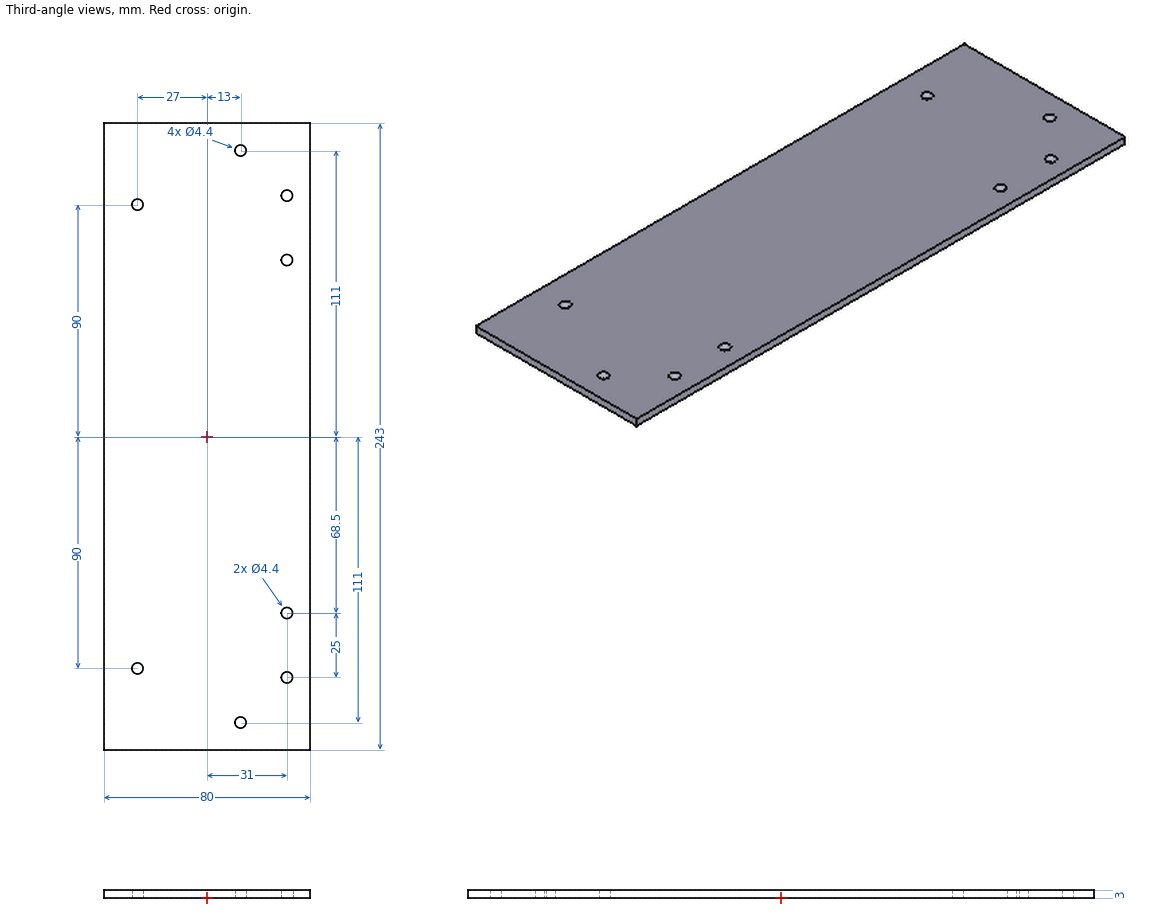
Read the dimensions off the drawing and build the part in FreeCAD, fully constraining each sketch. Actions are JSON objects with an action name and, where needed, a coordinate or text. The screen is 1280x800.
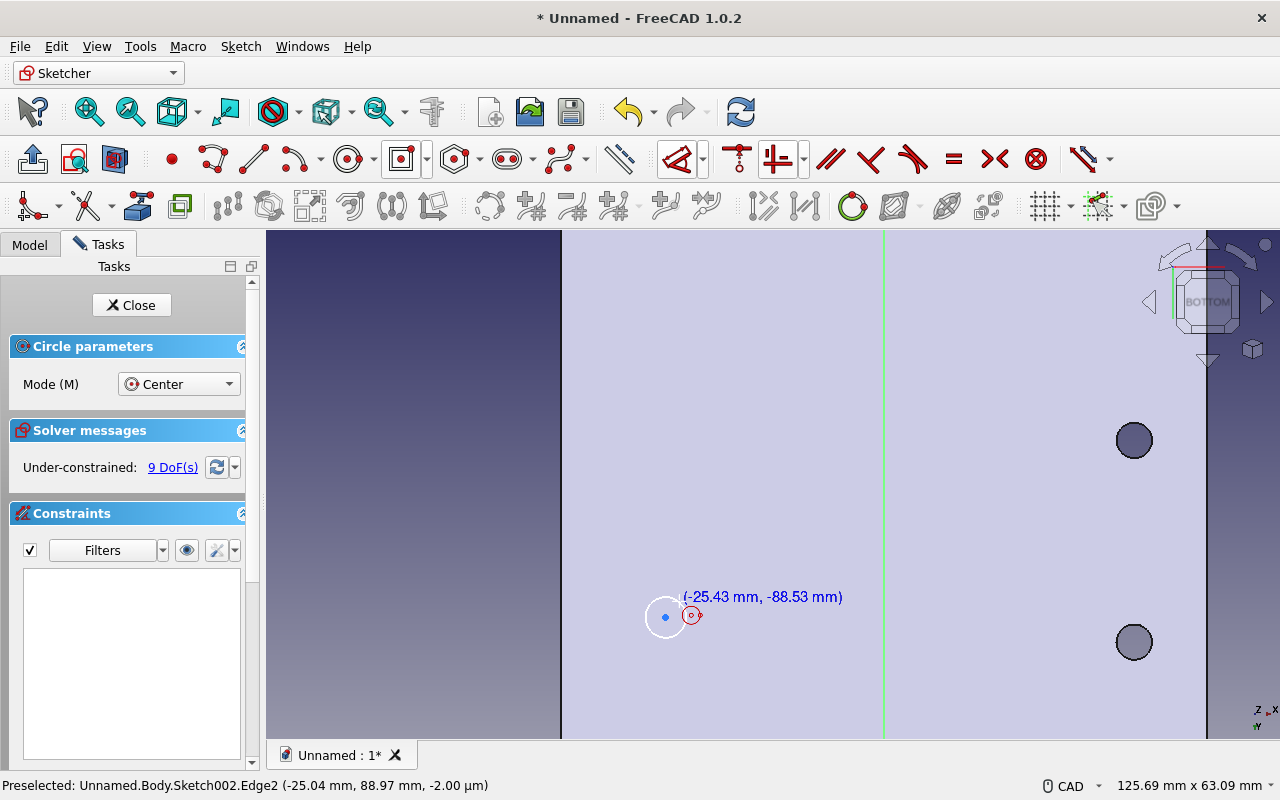
{"action": "scroll", "coordinate": [680, 603], "scroll_direction": "down", "scroll_amount": 9}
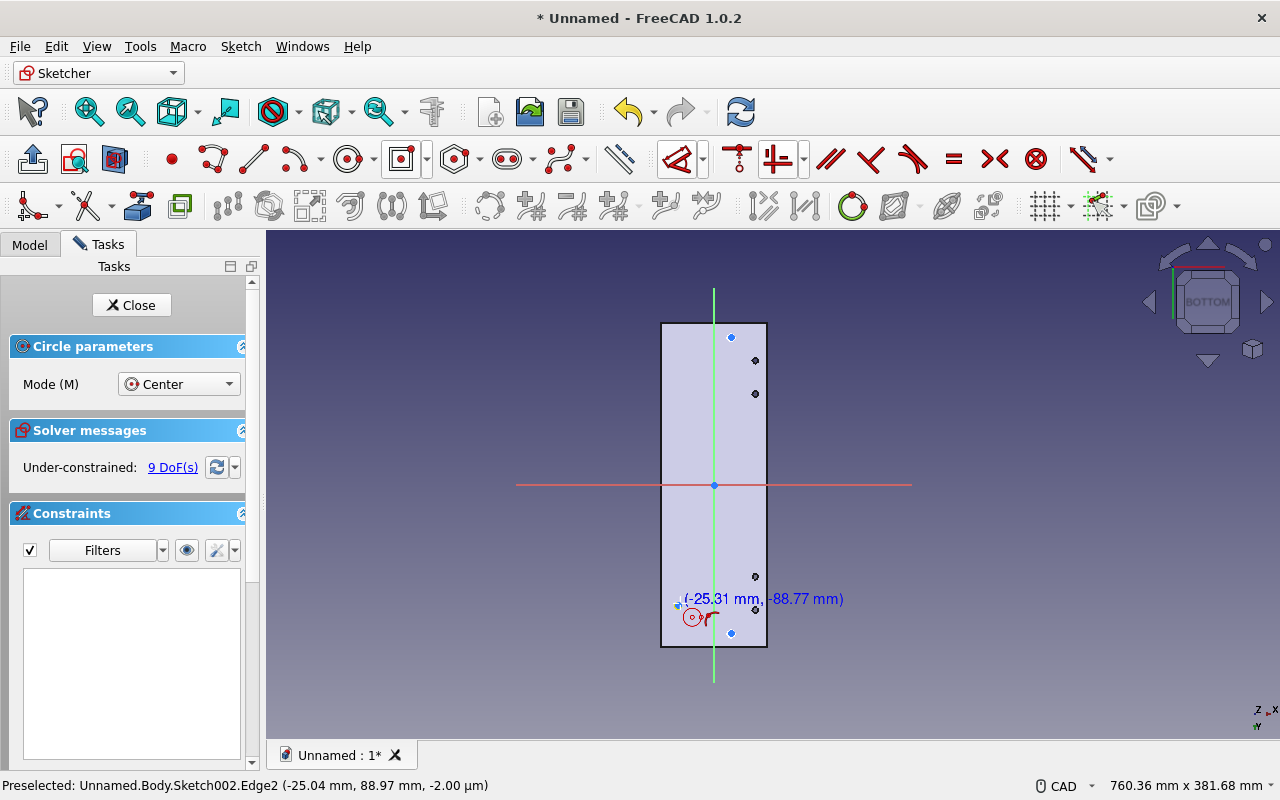
{"action": "scroll", "coordinate": [678, 365], "scroll_direction": "up", "scroll_amount": 11}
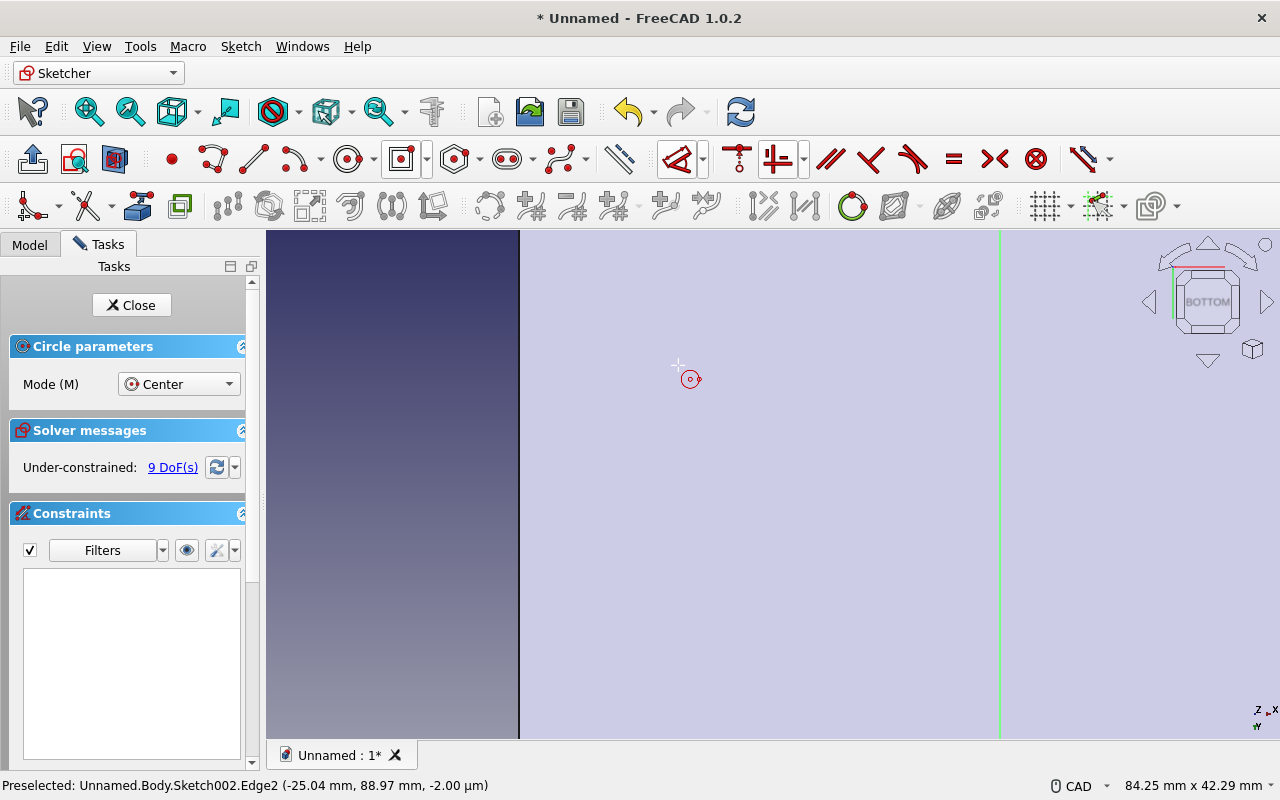
{"action": "scroll", "coordinate": [678, 364], "scroll_direction": "down", "scroll_amount": 11}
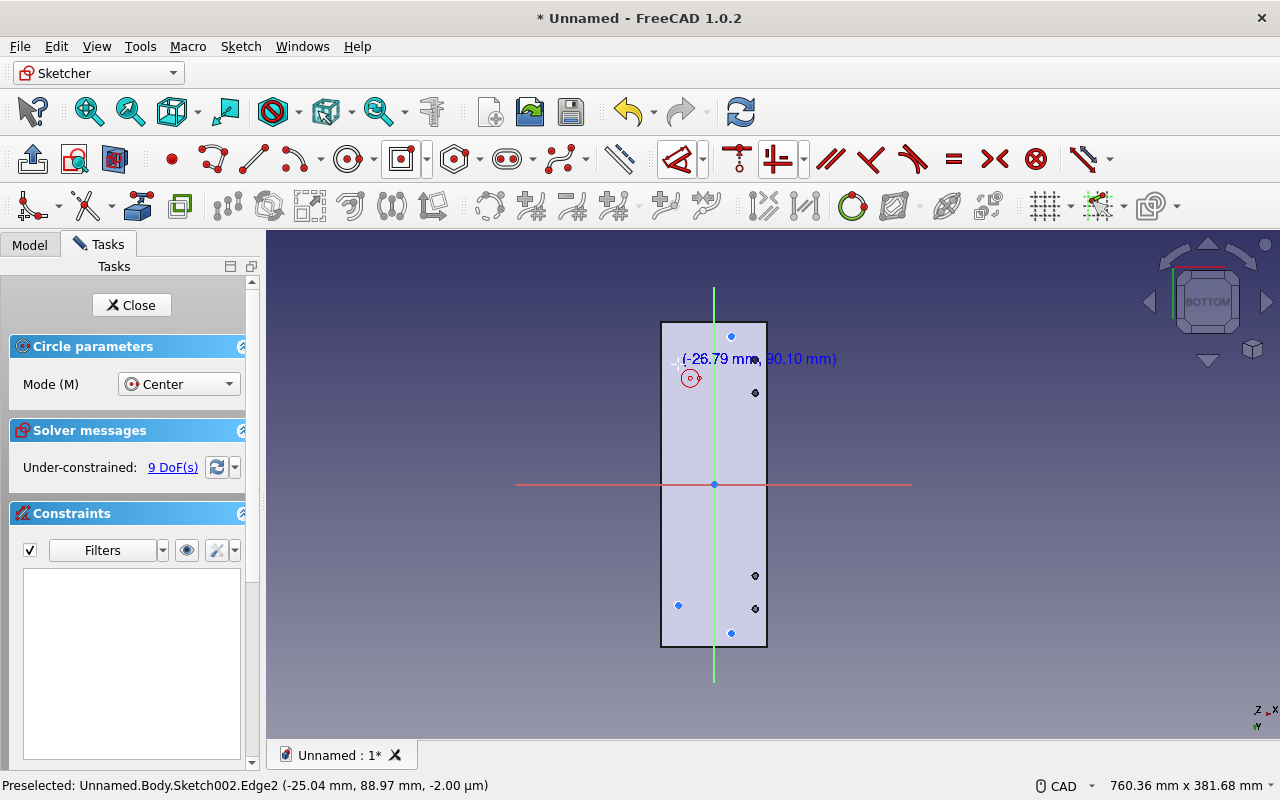
{"action": "left_click", "coordinate": [678, 364]}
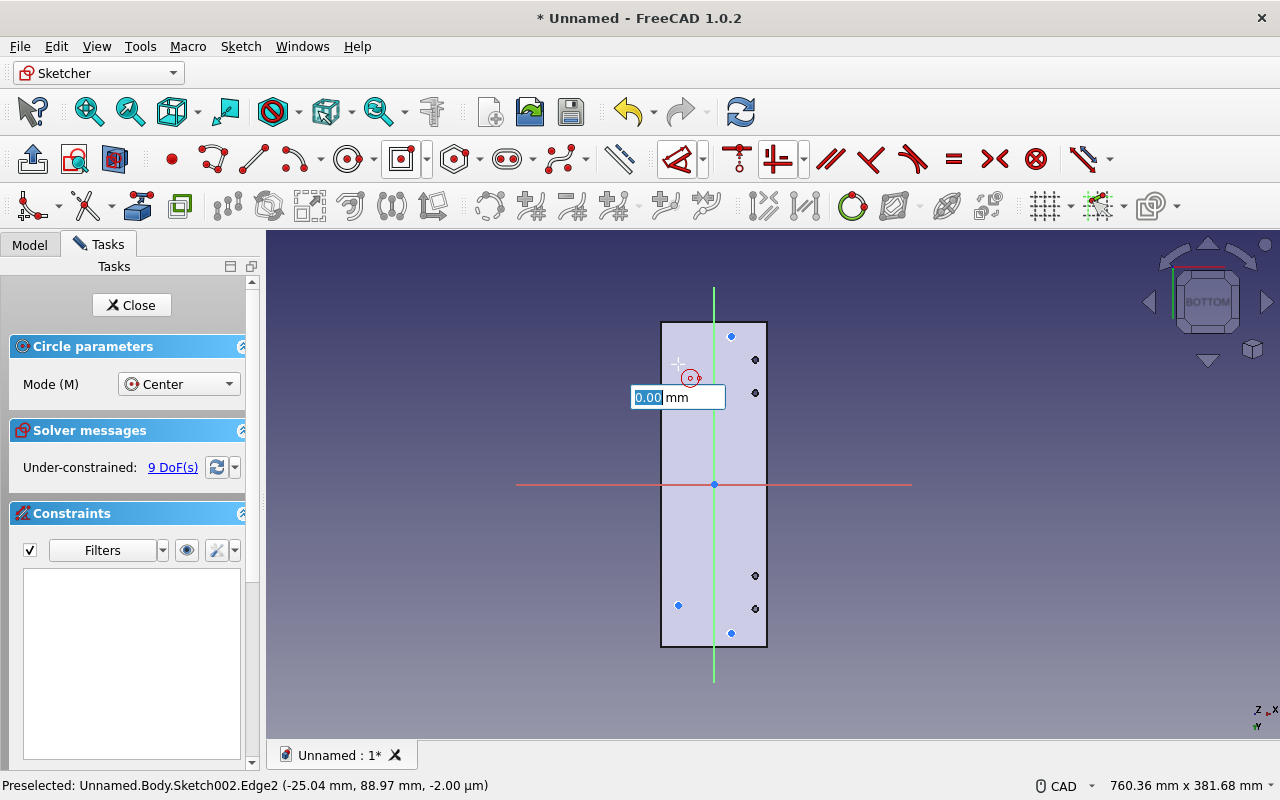
{"action": "scroll", "coordinate": [680, 362], "scroll_direction": "up", "scroll_amount": 9}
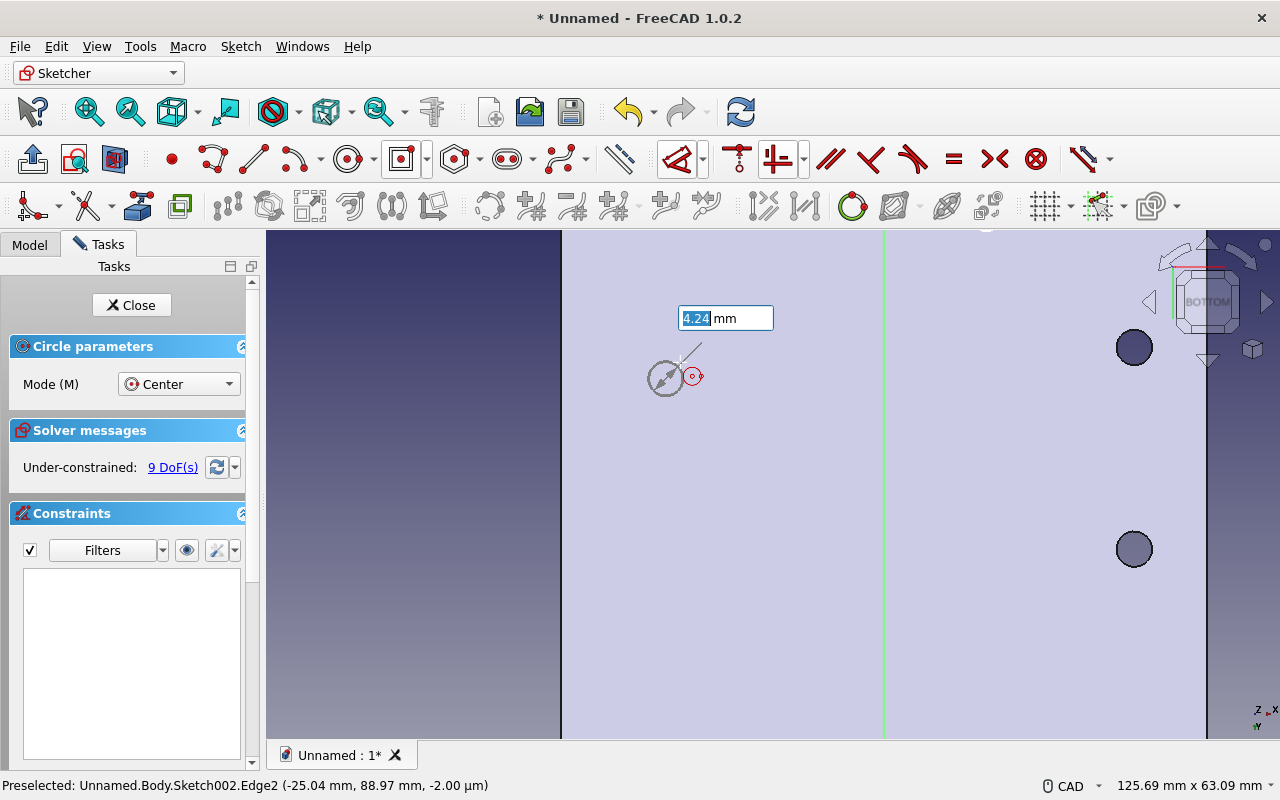
{"action": "left_click", "coordinate": [679, 363]}
{"action": "key", "text": "Escape"}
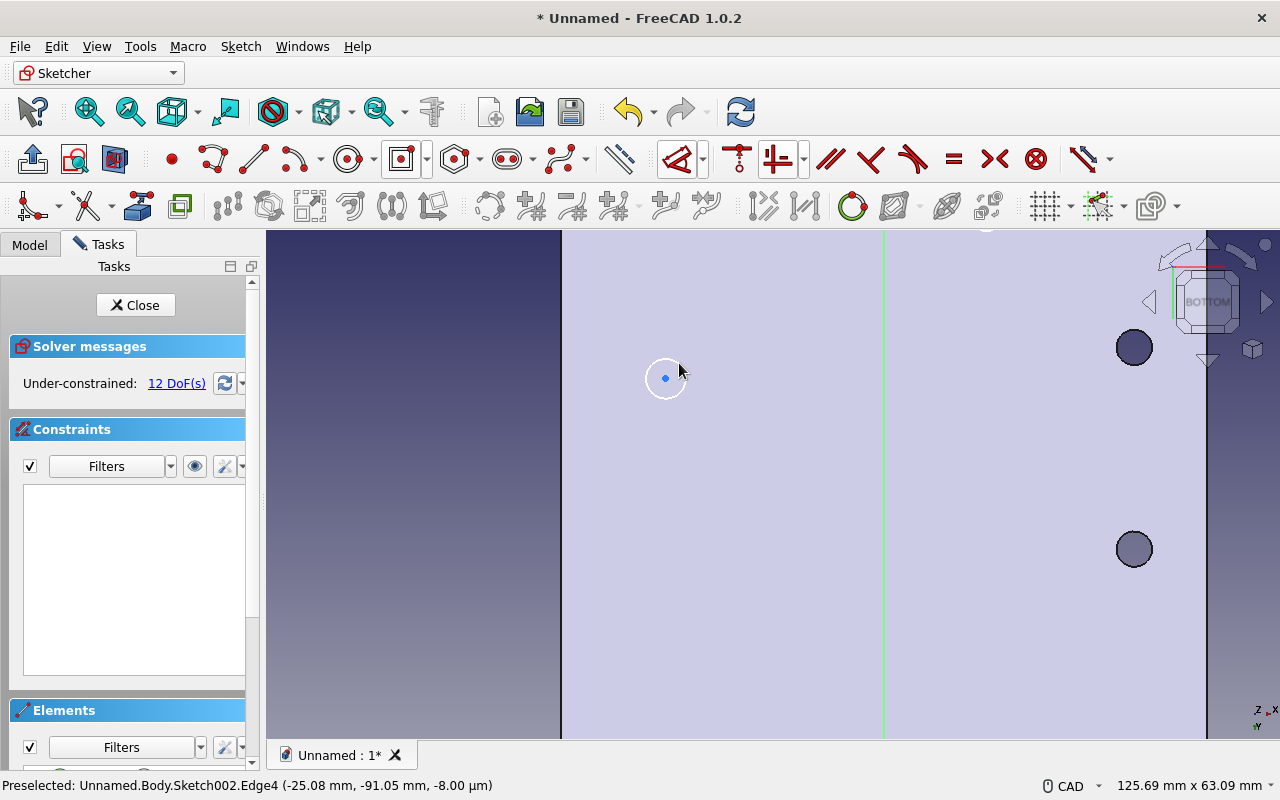
{"action": "scroll", "coordinate": [680, 362], "scroll_direction": "down", "scroll_amount": 9}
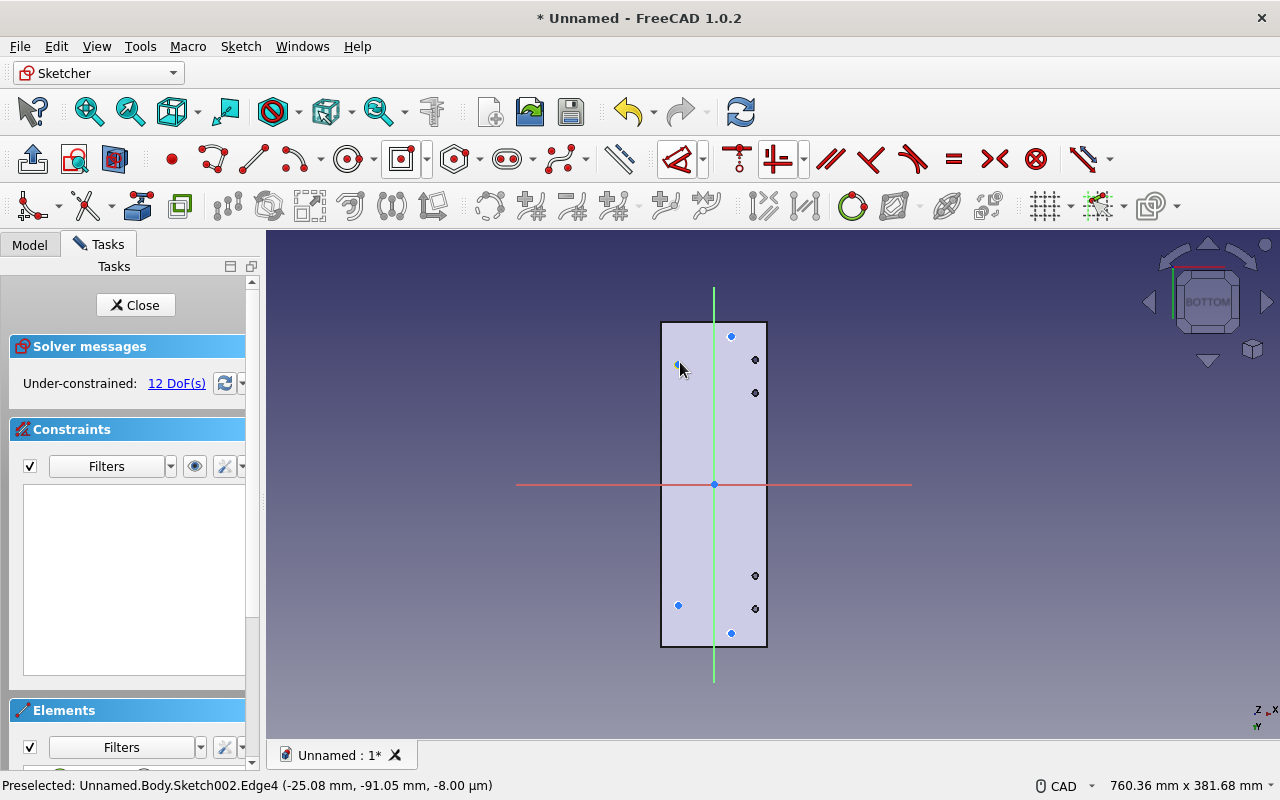
{"action": "scroll", "coordinate": [734, 631], "scroll_direction": "up", "scroll_amount": 7}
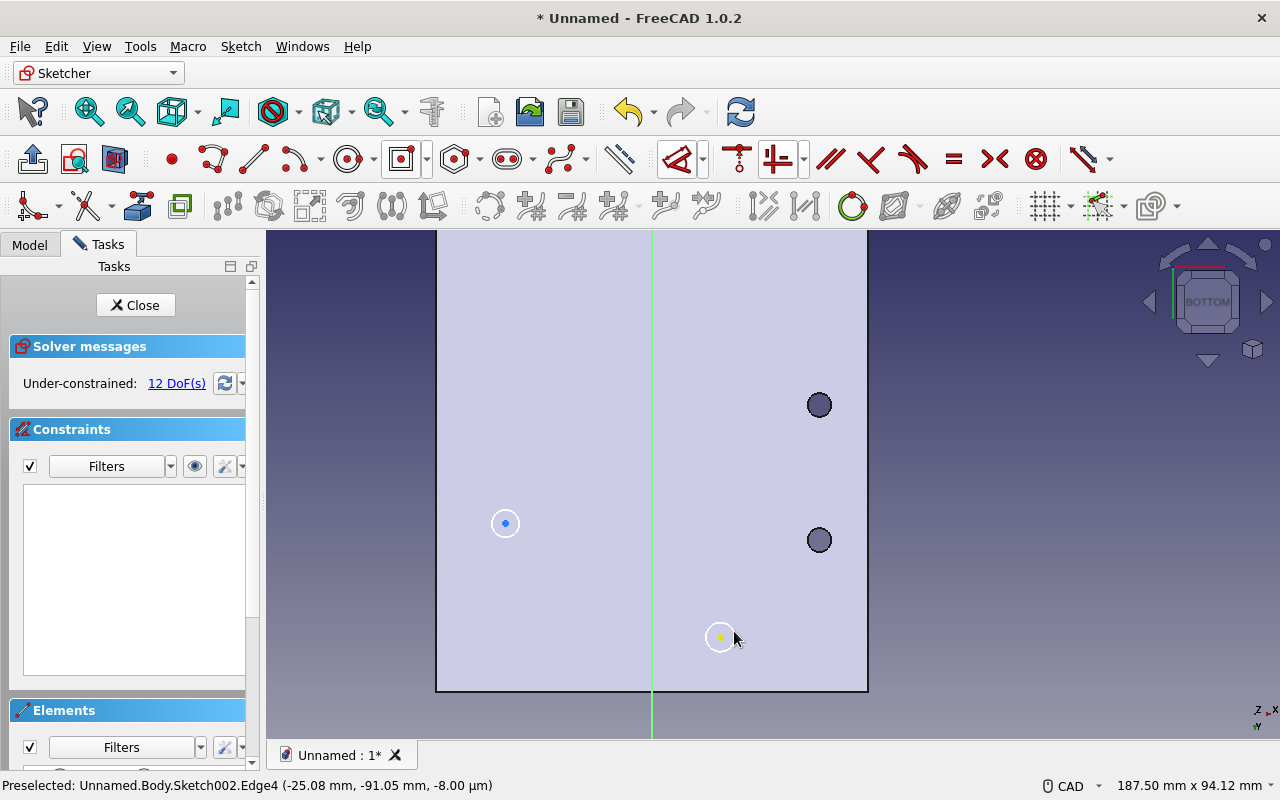
{"action": "left_click", "coordinate": [731, 627]}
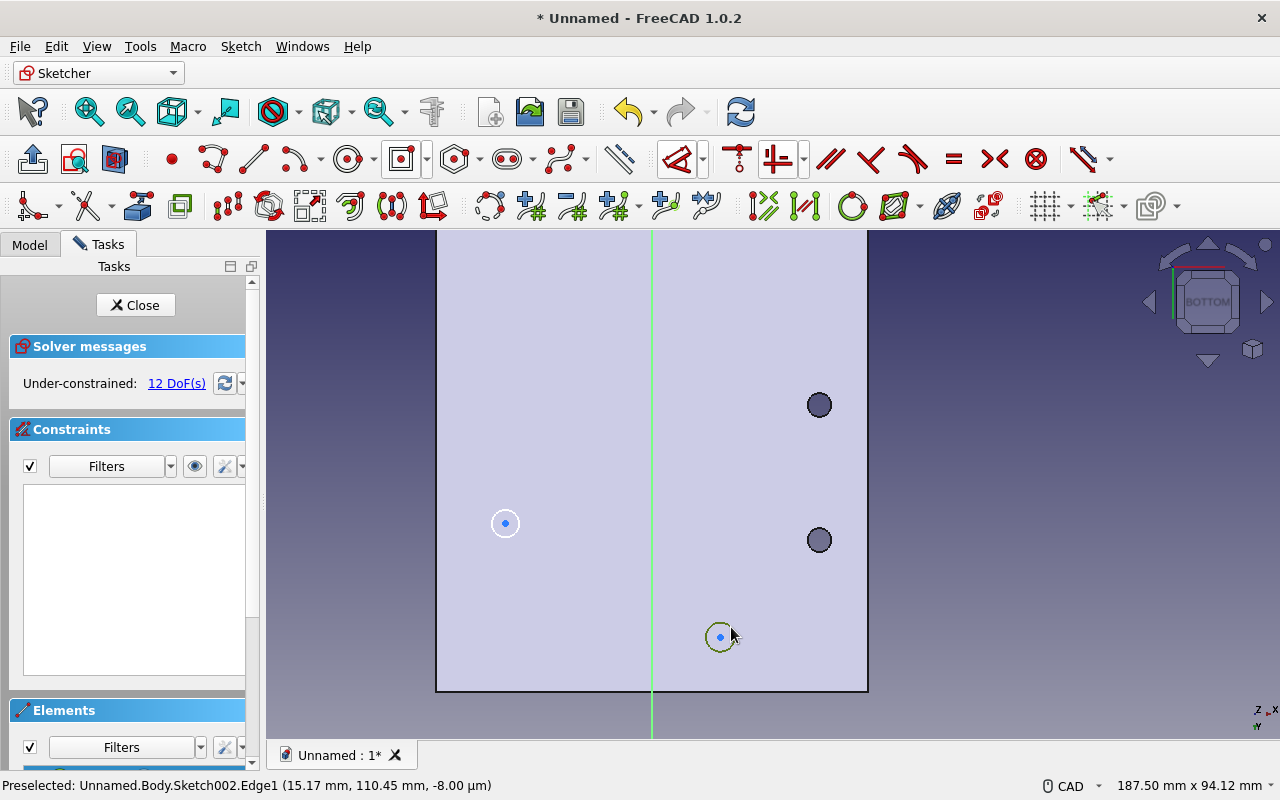
{"action": "scroll", "coordinate": [734, 632], "scroll_direction": "down", "scroll_amount": 7}